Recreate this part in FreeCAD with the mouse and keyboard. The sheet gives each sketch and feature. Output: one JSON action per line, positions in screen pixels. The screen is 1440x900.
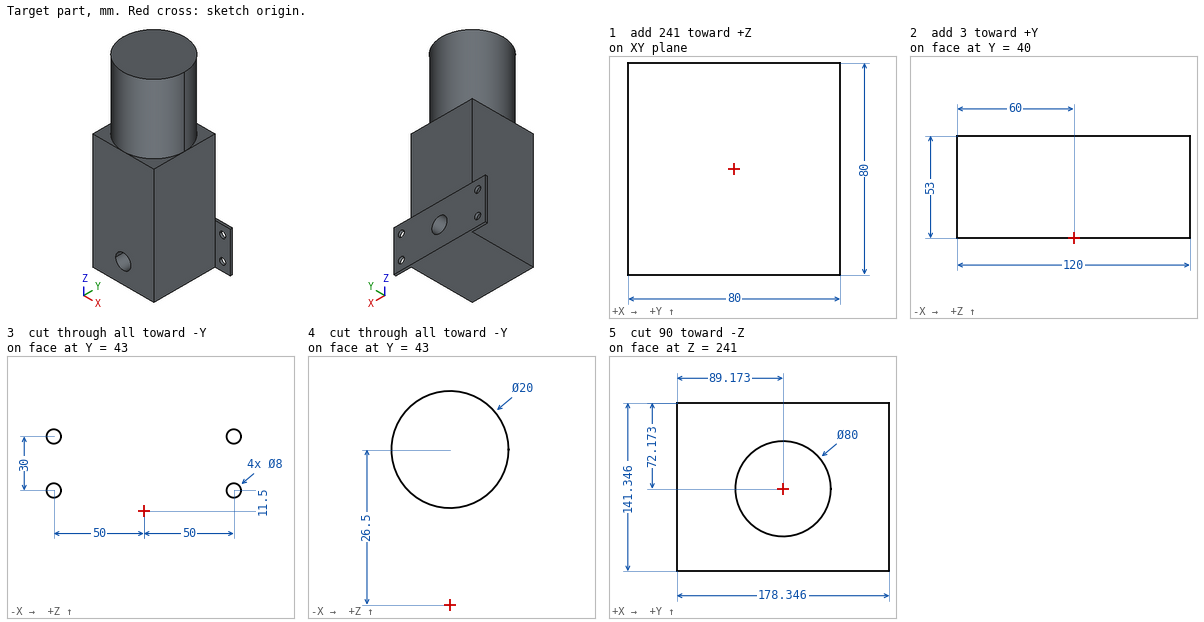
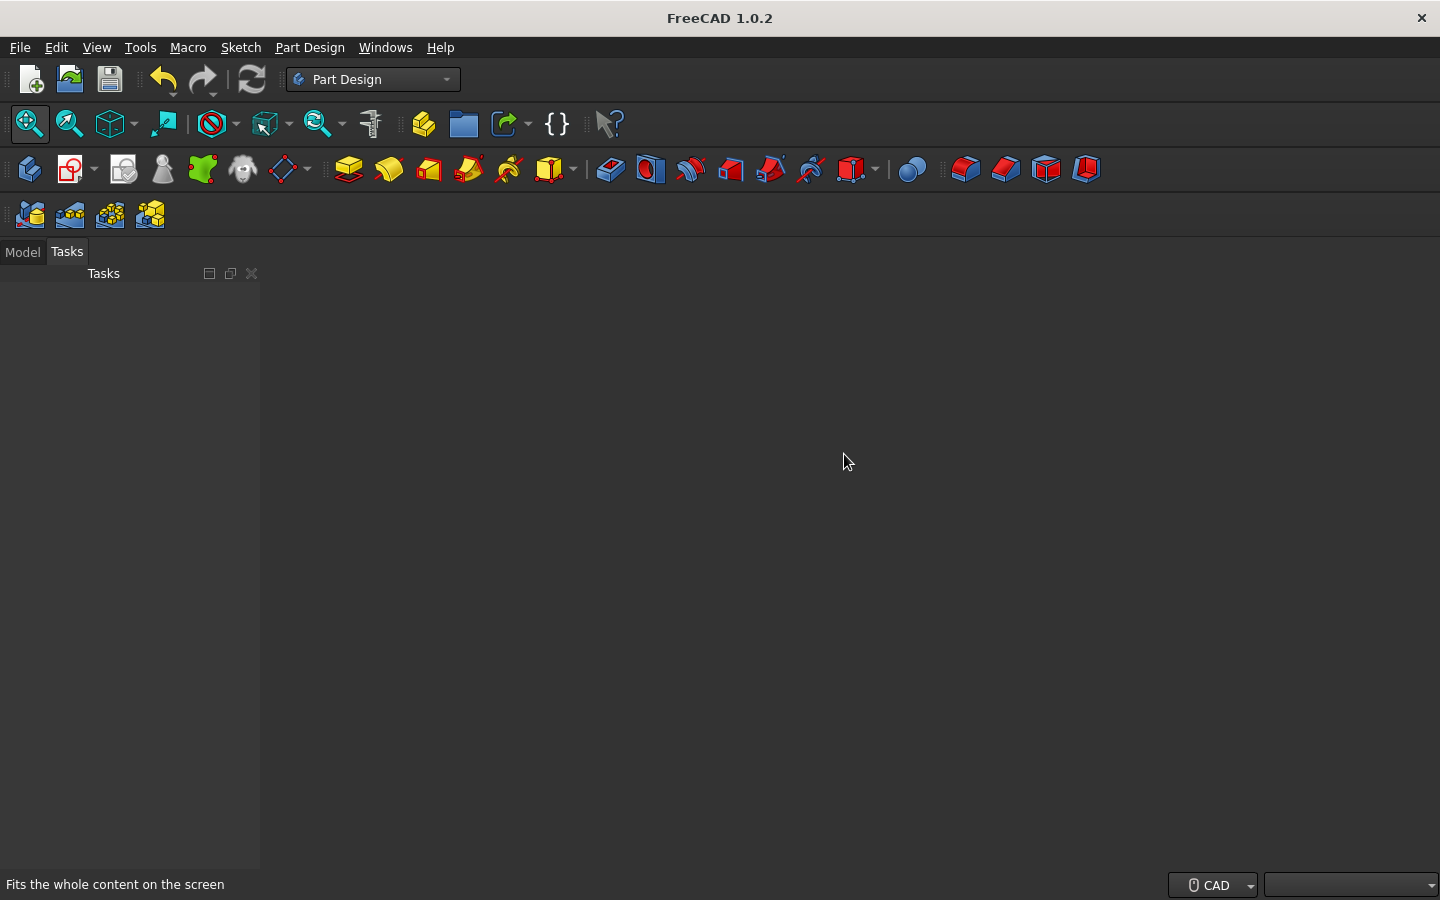
{"action": "left_click", "coordinate": [30, 80]}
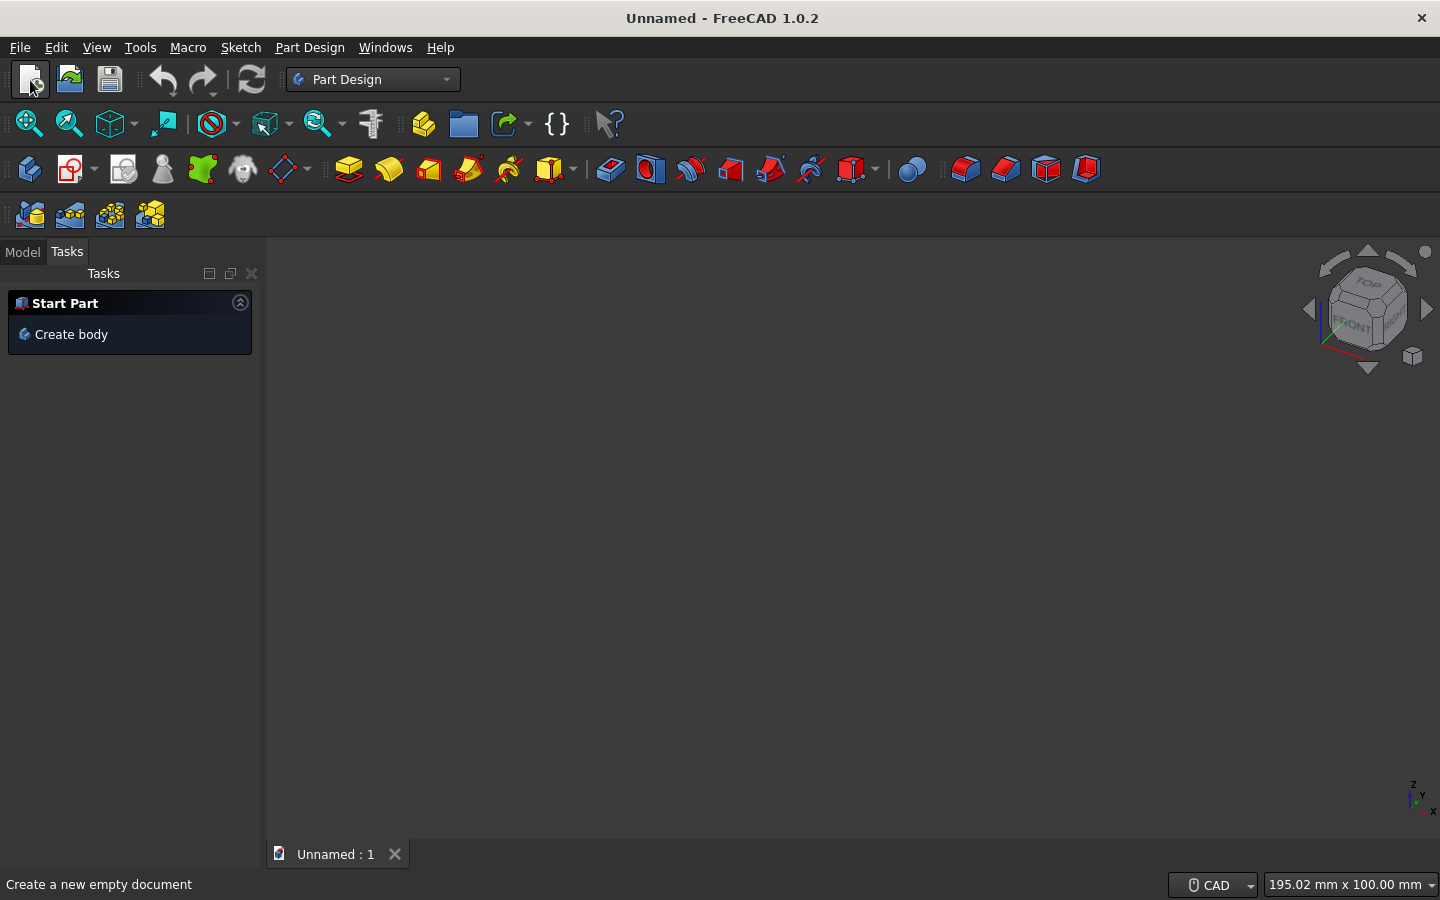
{"action": "left_click", "coordinate": [70, 170]}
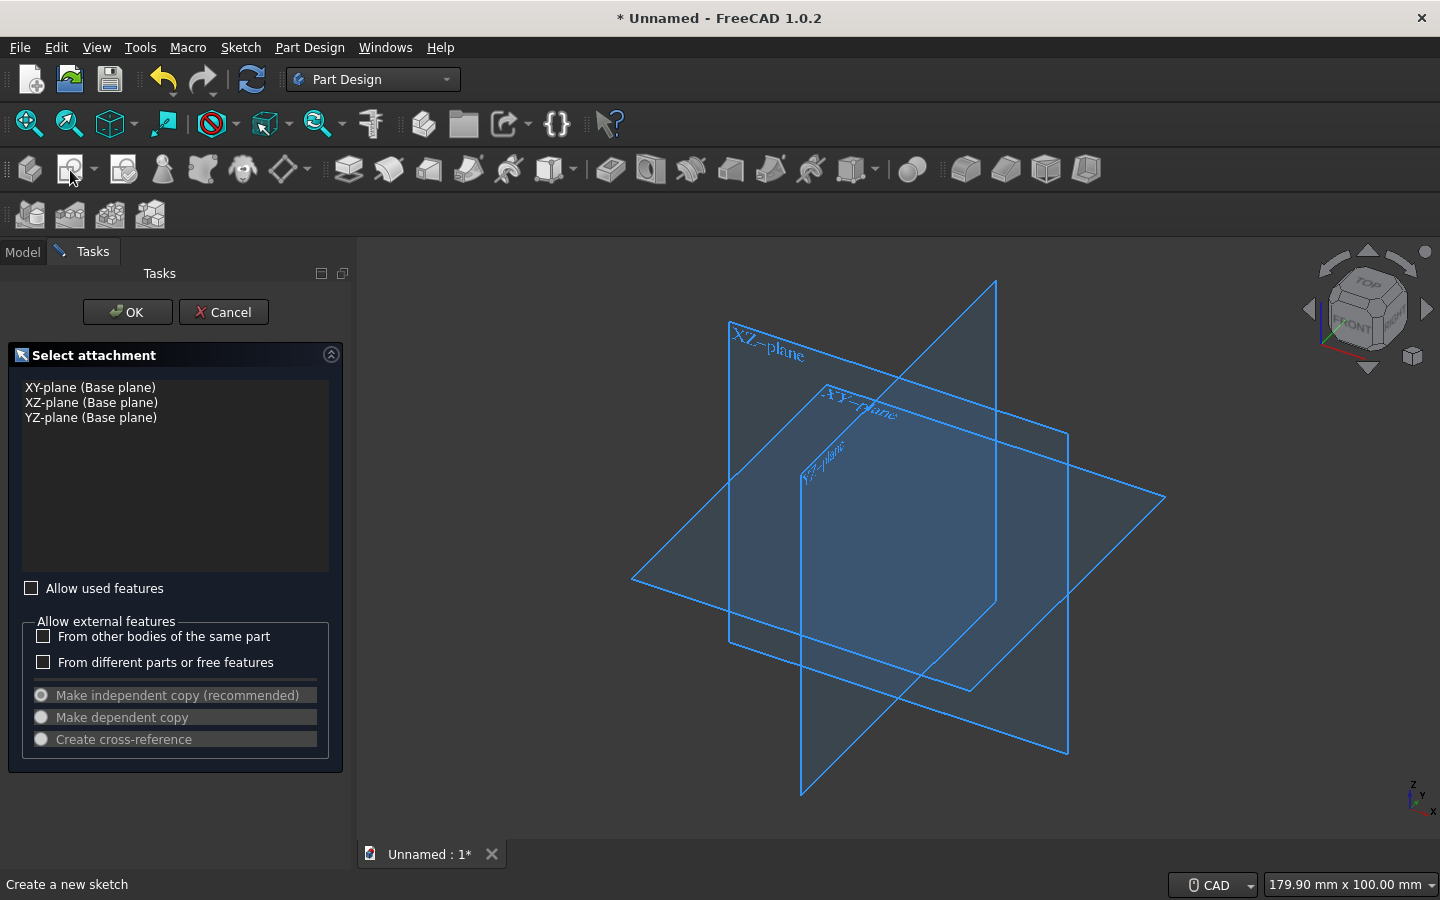
{"action": "left_click", "coordinate": [82, 388]}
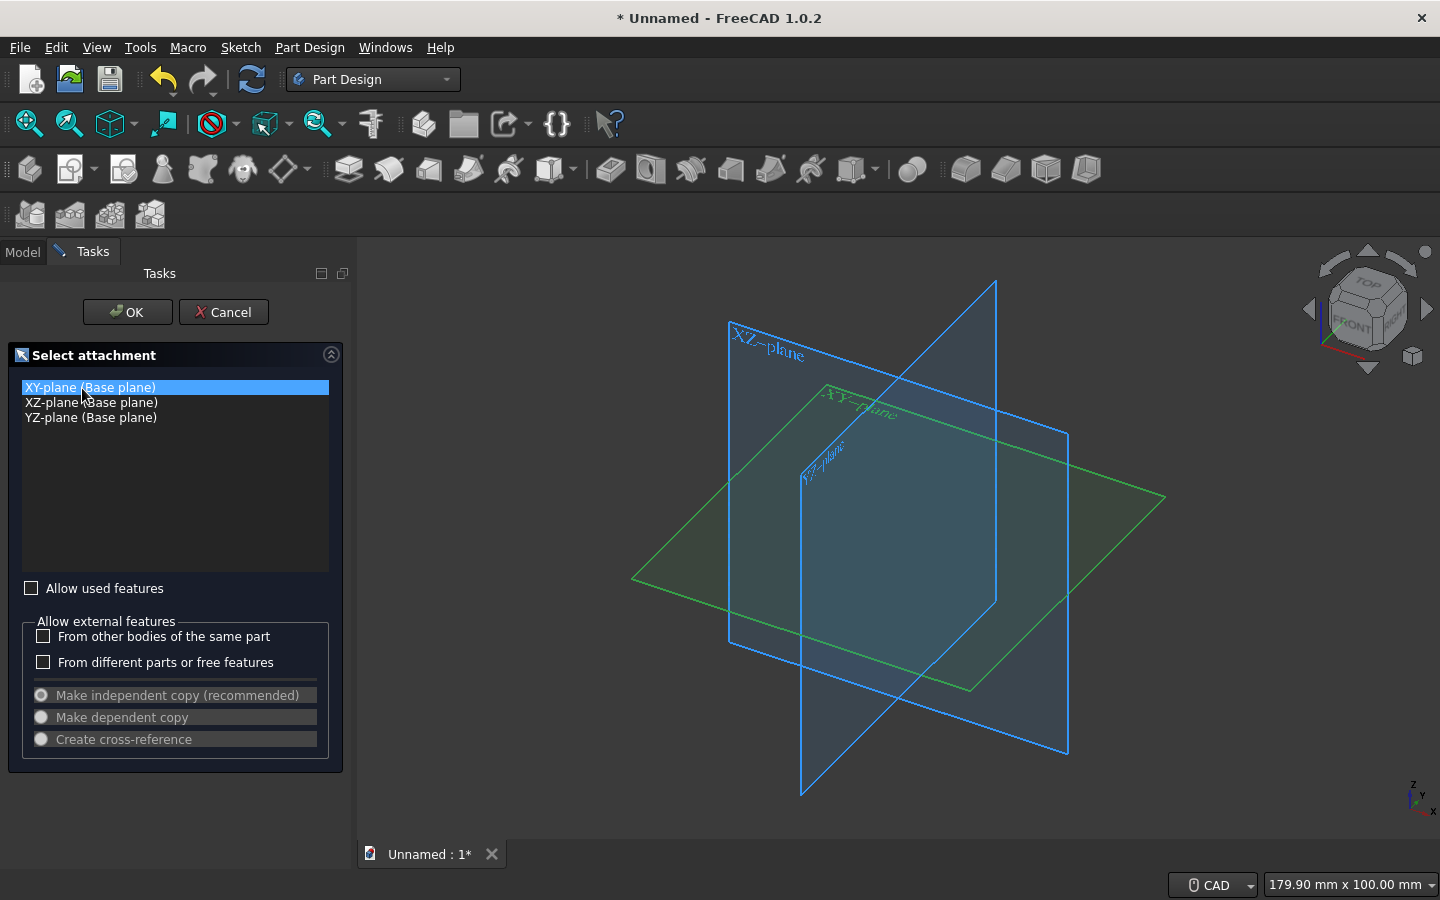
{"action": "left_click", "coordinate": [128, 312]}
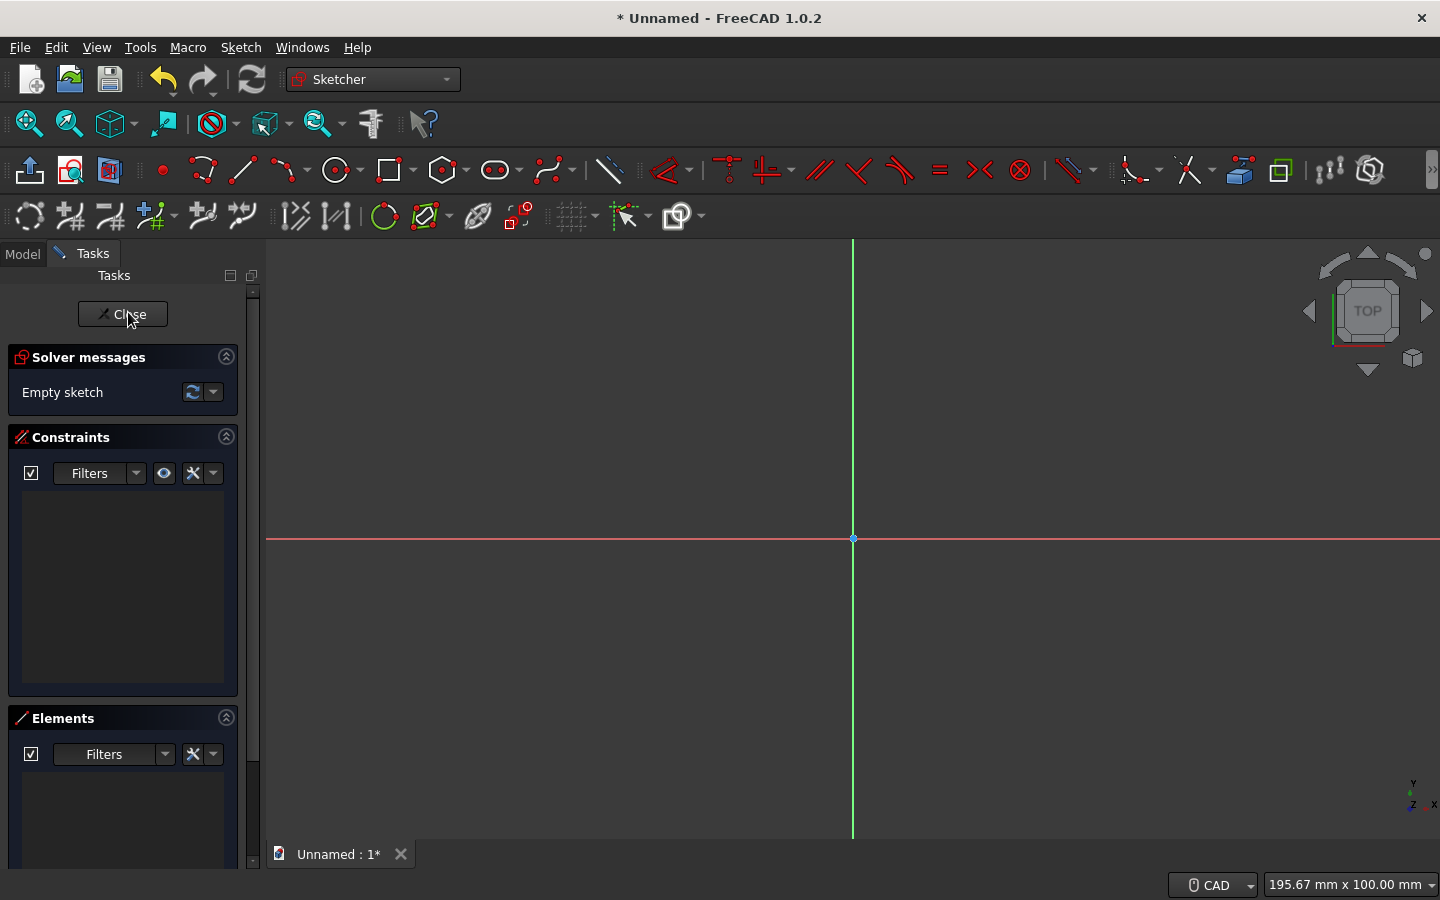
{"action": "key", "text": "g v"}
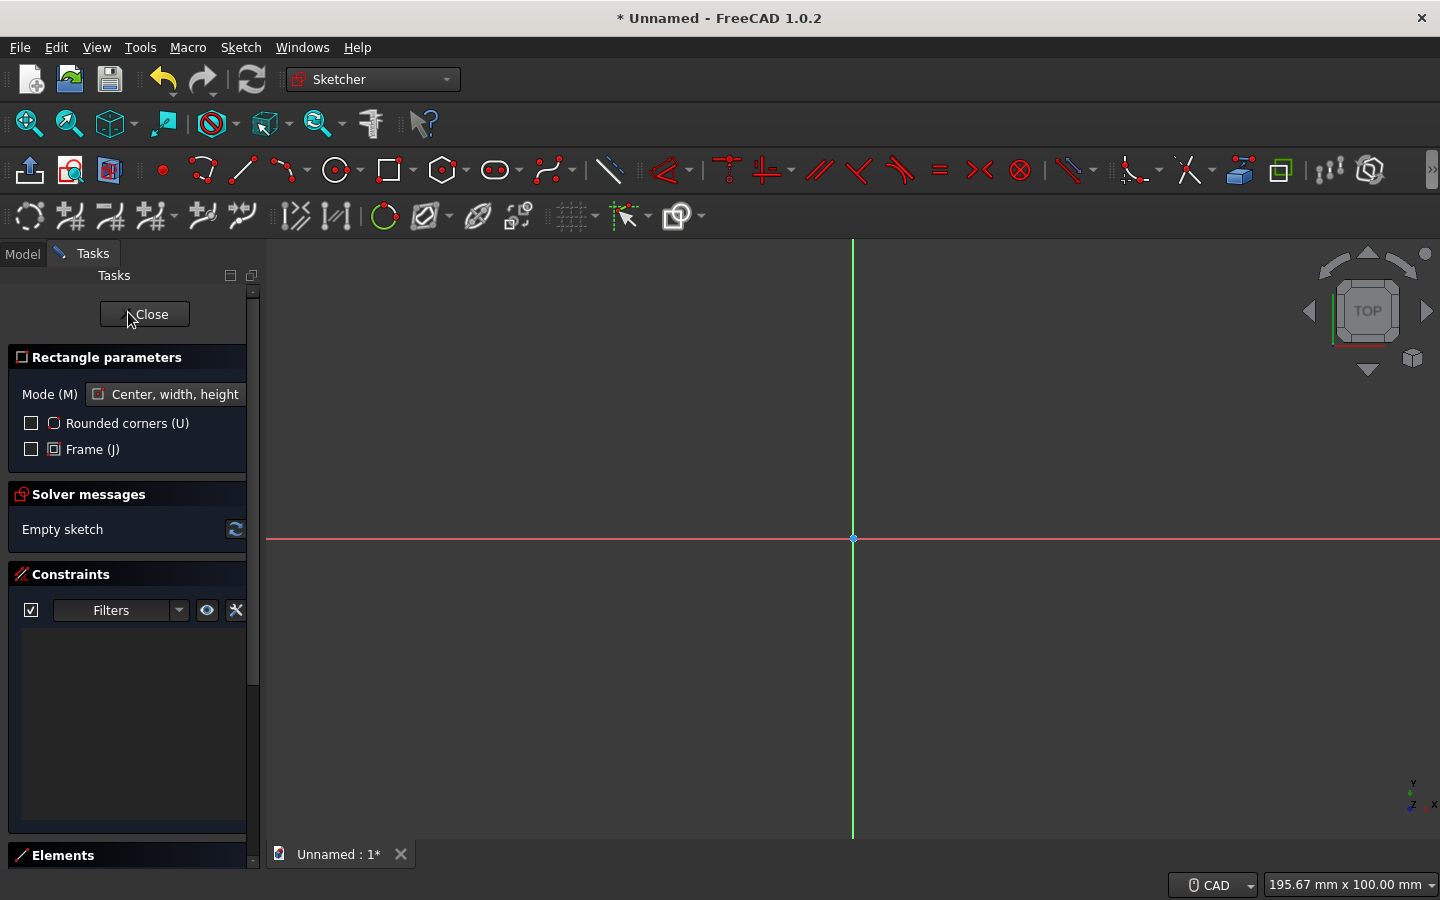
{"action": "left_click", "coordinate": [853, 539]}
{"action": "left_click", "coordinate": [1093, 299]}
{"action": "key", "text": "Escape"}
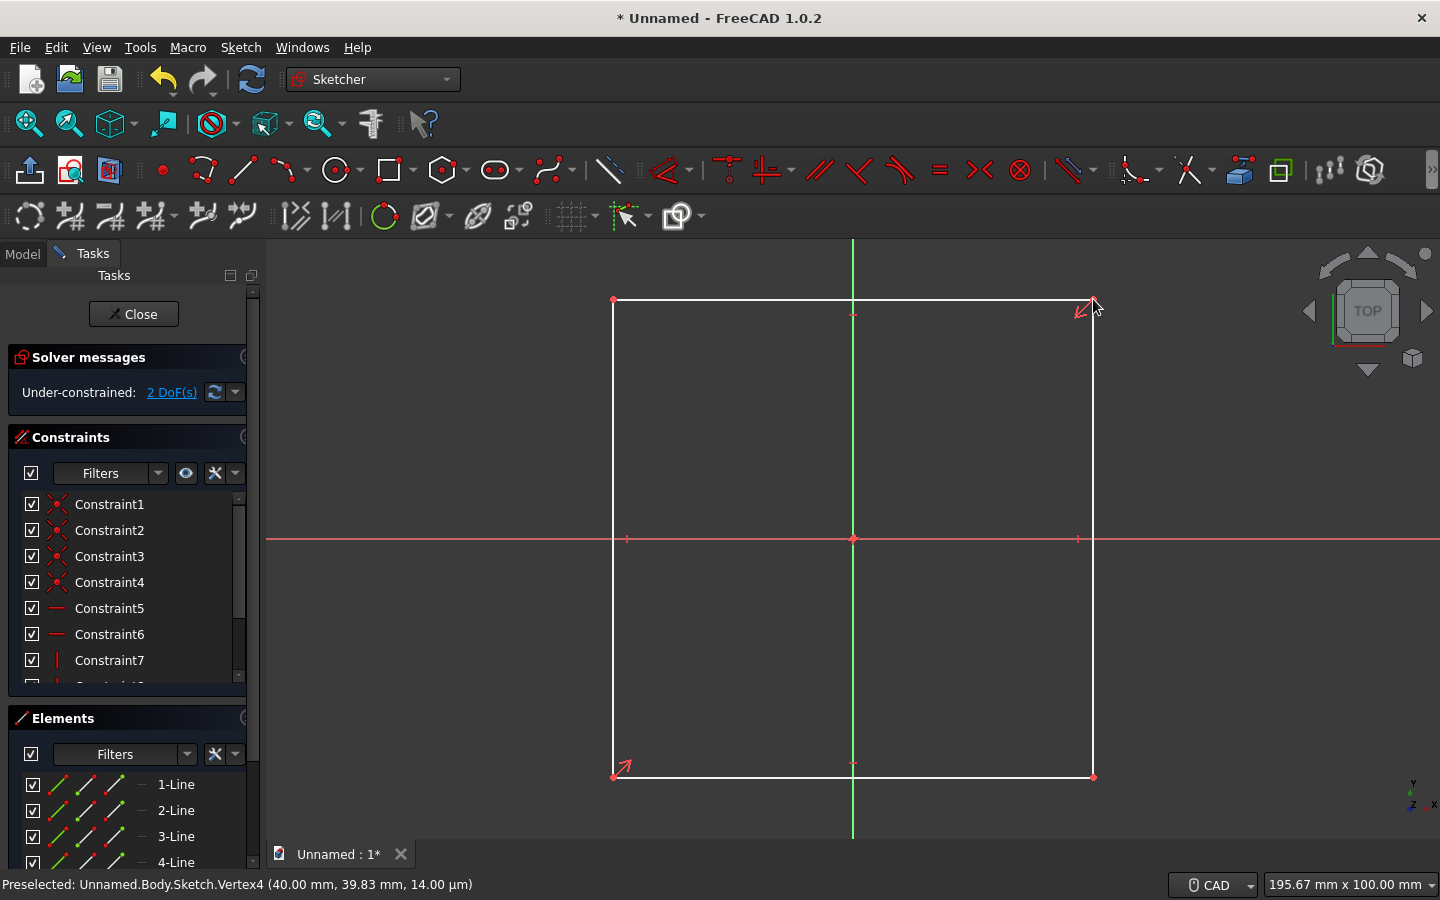
{"action": "left_click", "coordinate": [664, 170]}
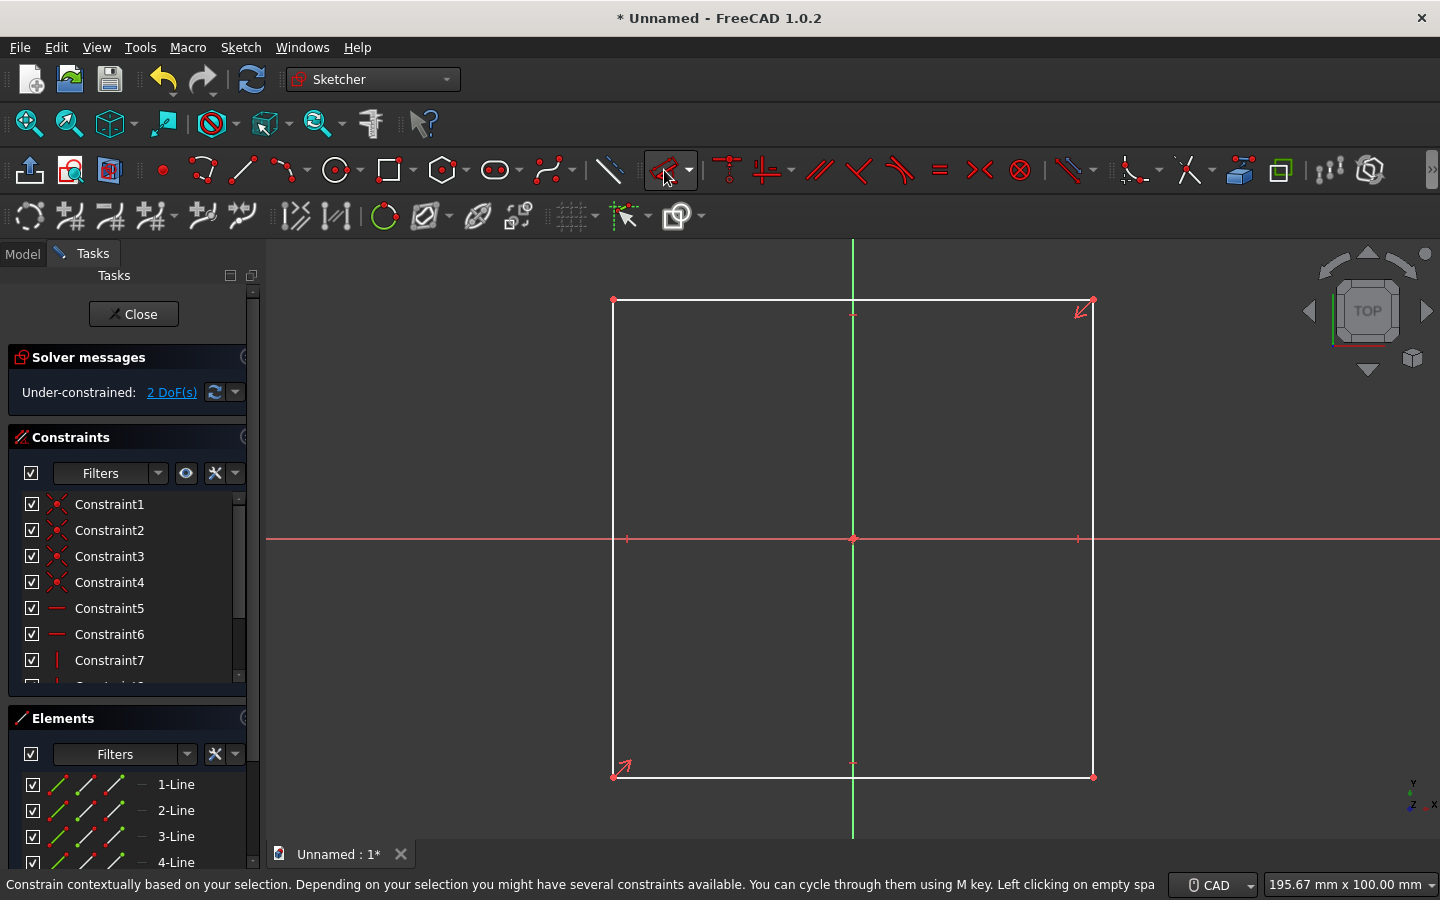
{"action": "left_click", "coordinate": [757, 778]}
{"action": "left_click", "coordinate": [743, 744]}